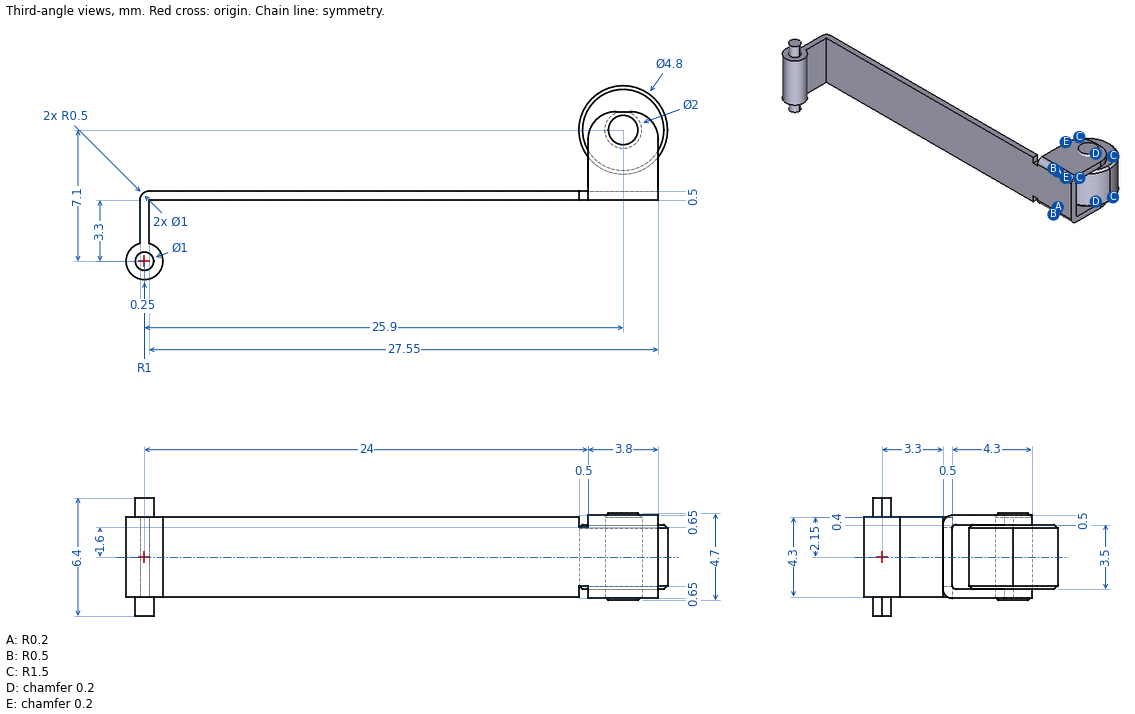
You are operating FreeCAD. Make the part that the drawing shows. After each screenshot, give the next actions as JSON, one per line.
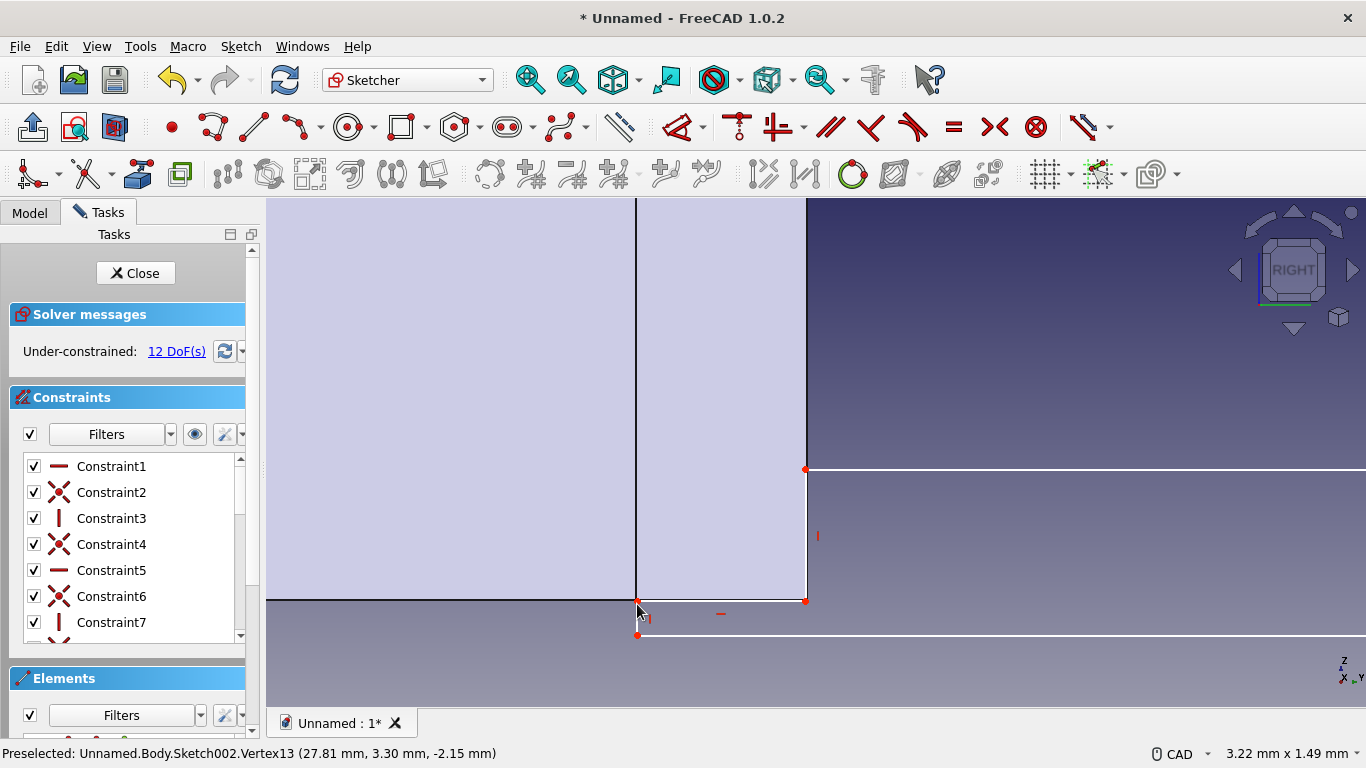
{"action": "scroll", "coordinate": [711, 601], "scroll_direction": "down", "scroll_amount": 8}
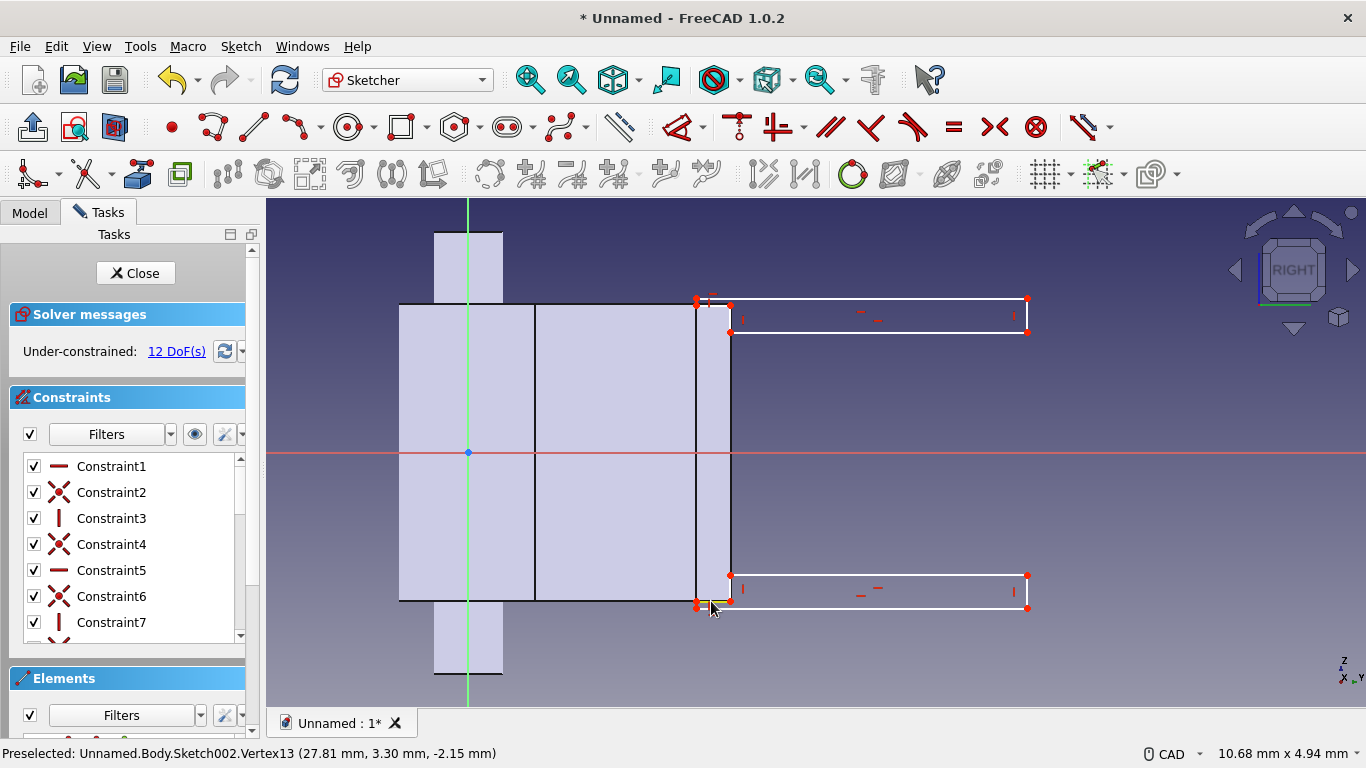
{"action": "scroll", "coordinate": [696, 306], "scroll_direction": "up", "scroll_amount": 3}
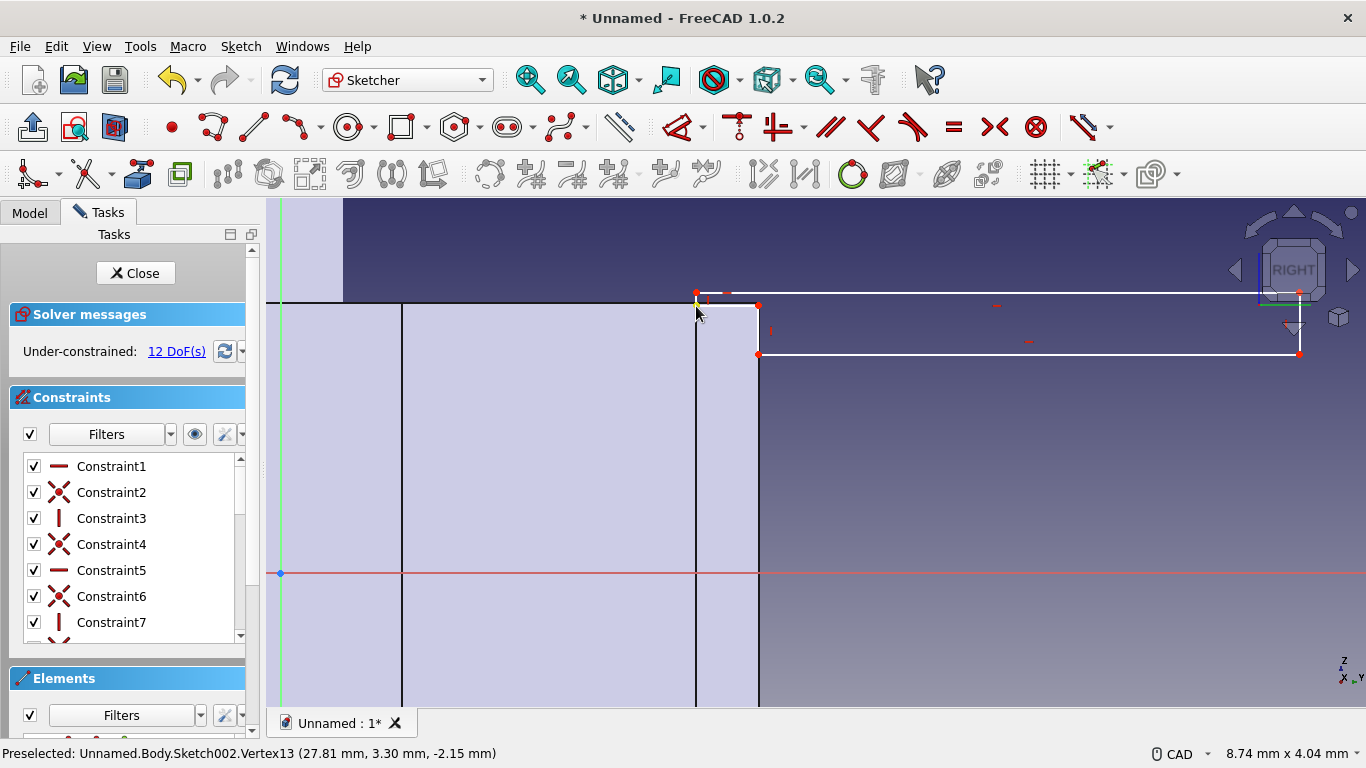
{"action": "left_click", "coordinate": [696, 306]}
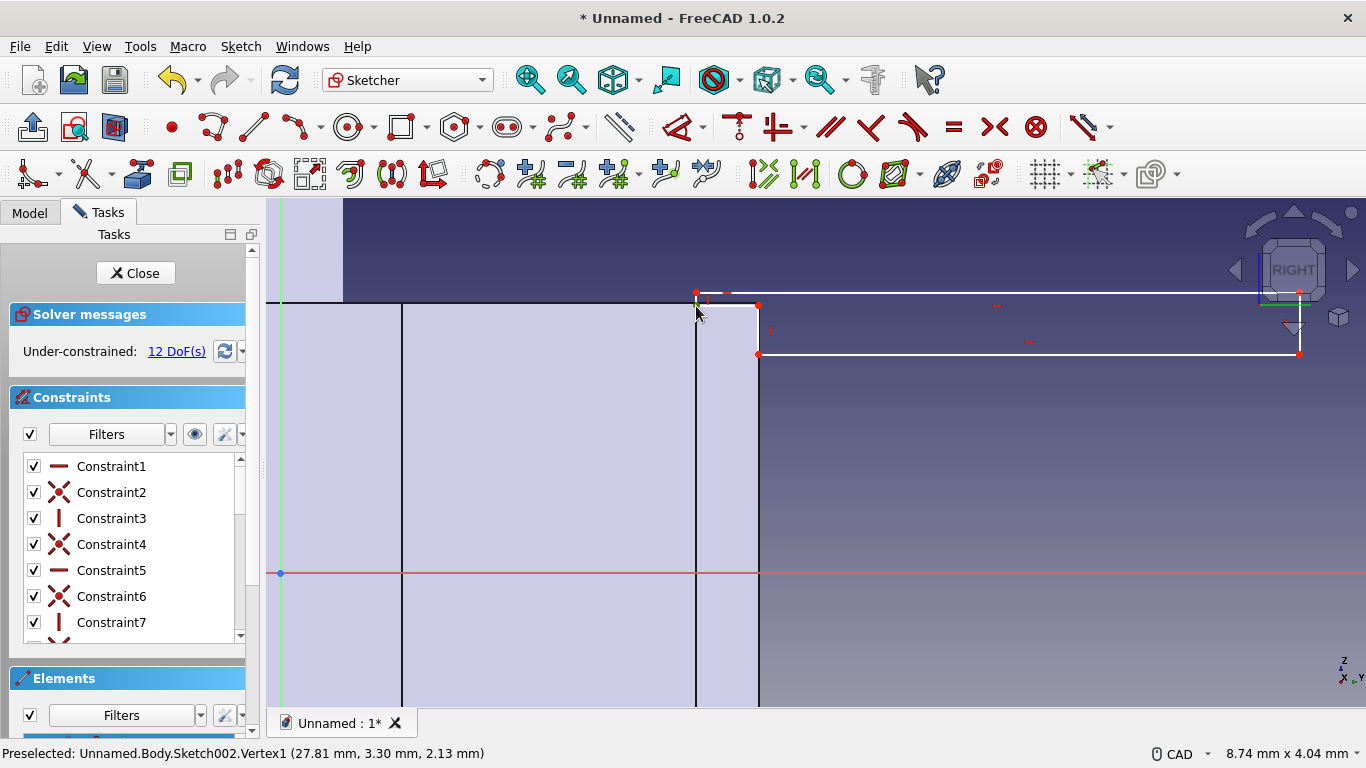
{"action": "scroll", "coordinate": [695, 305], "scroll_direction": "down", "scroll_amount": 3}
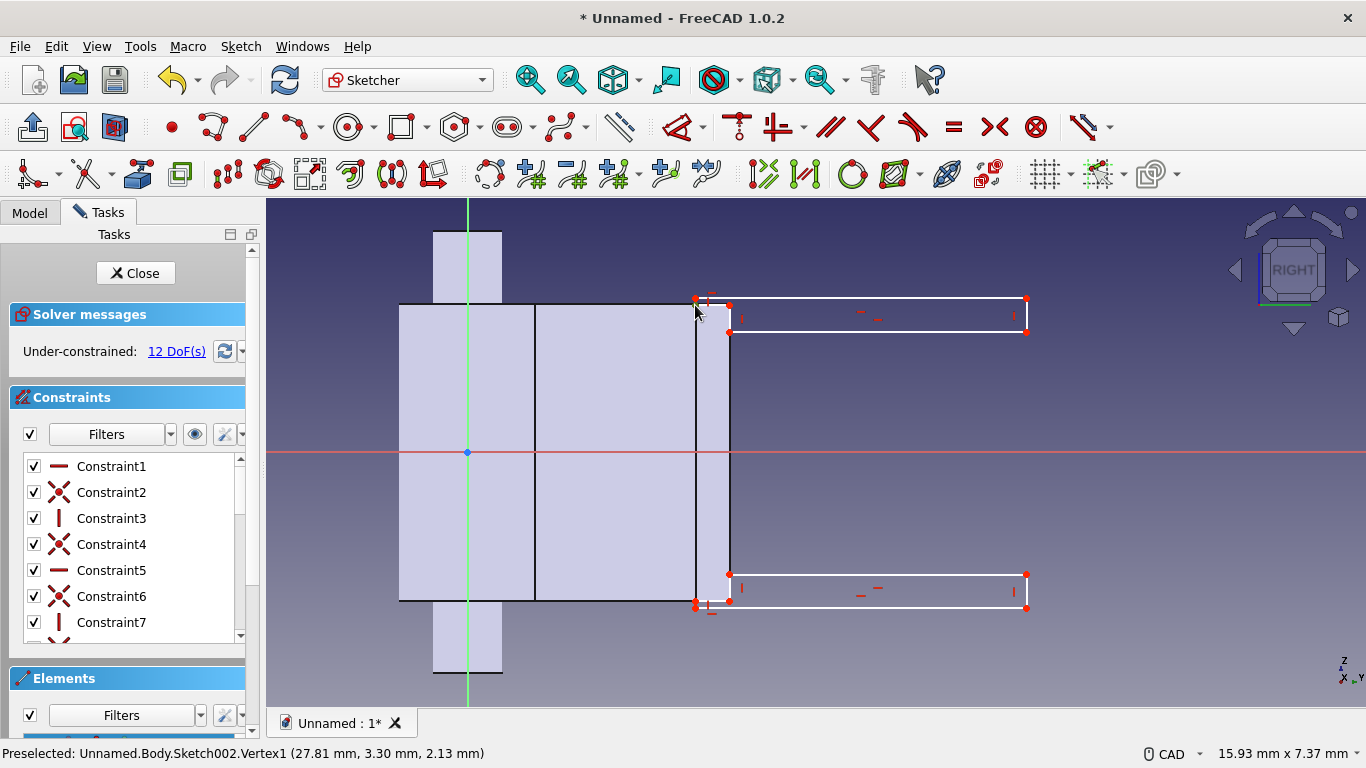
{"action": "scroll", "coordinate": [696, 601], "scroll_direction": "up", "scroll_amount": 3}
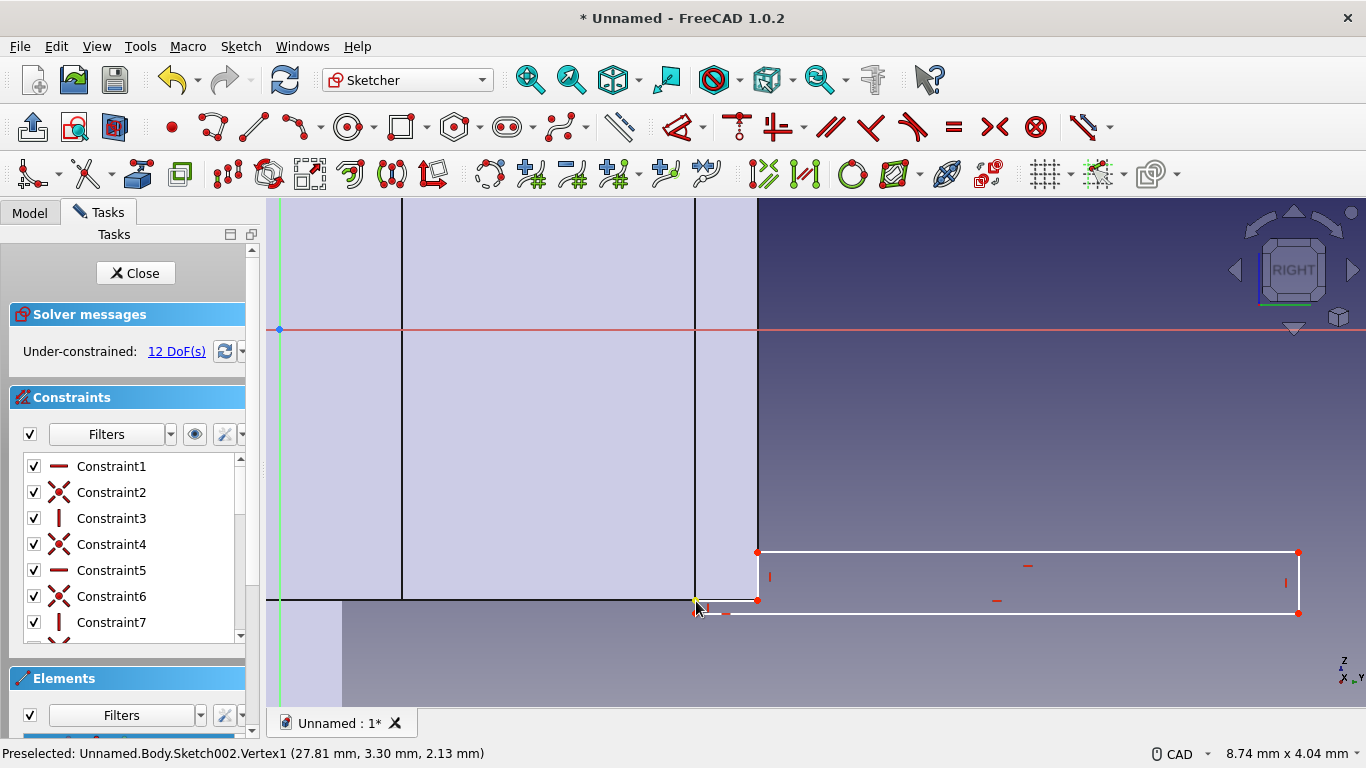
{"action": "left_click", "coordinate": [696, 601]}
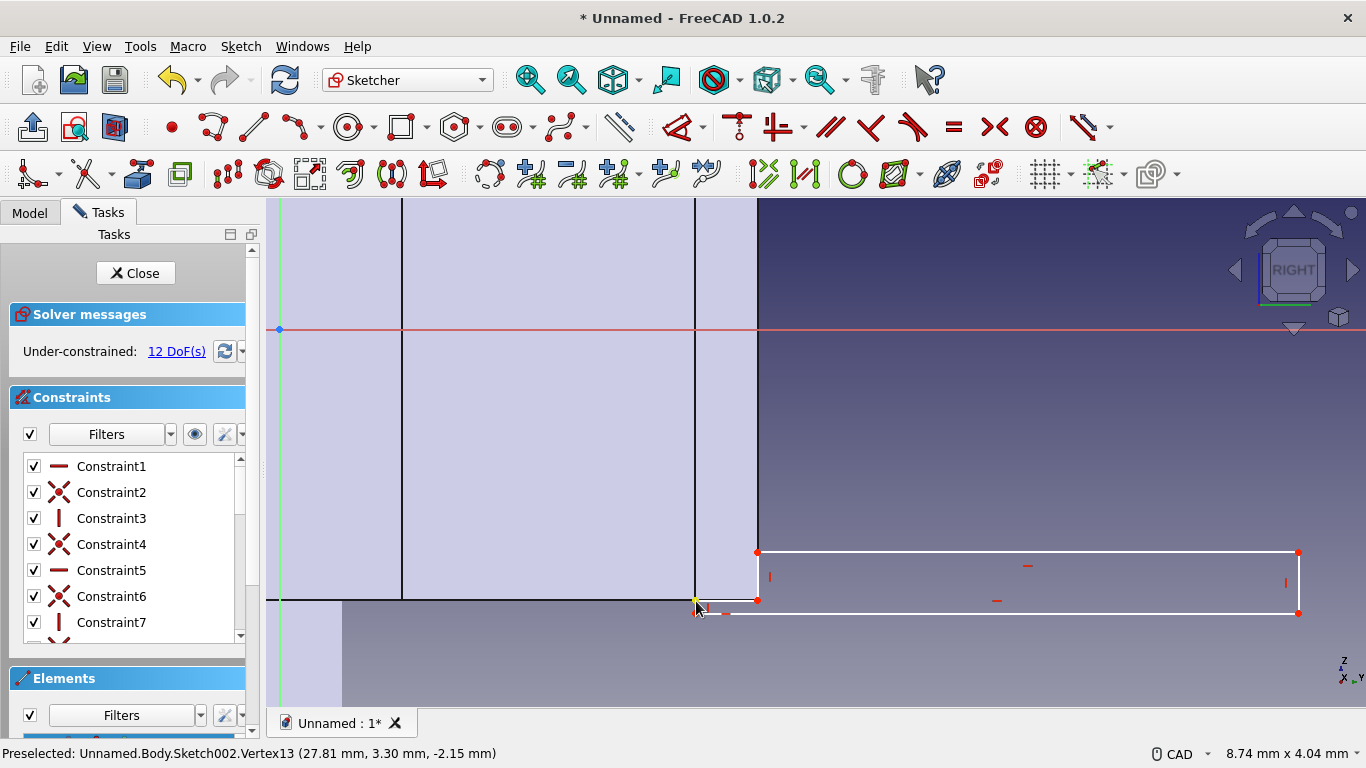
{"action": "left_click", "coordinate": [359, 330]}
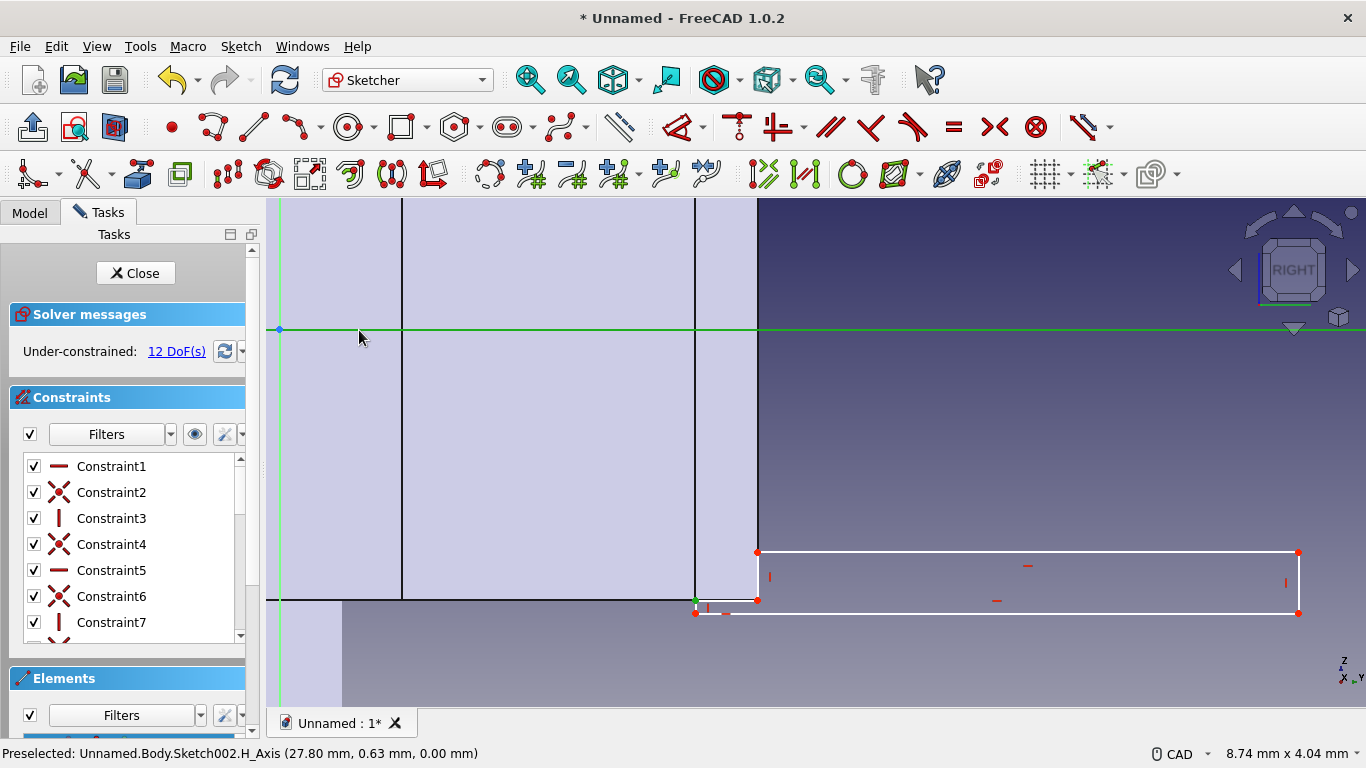
{"action": "key", "text": "s"}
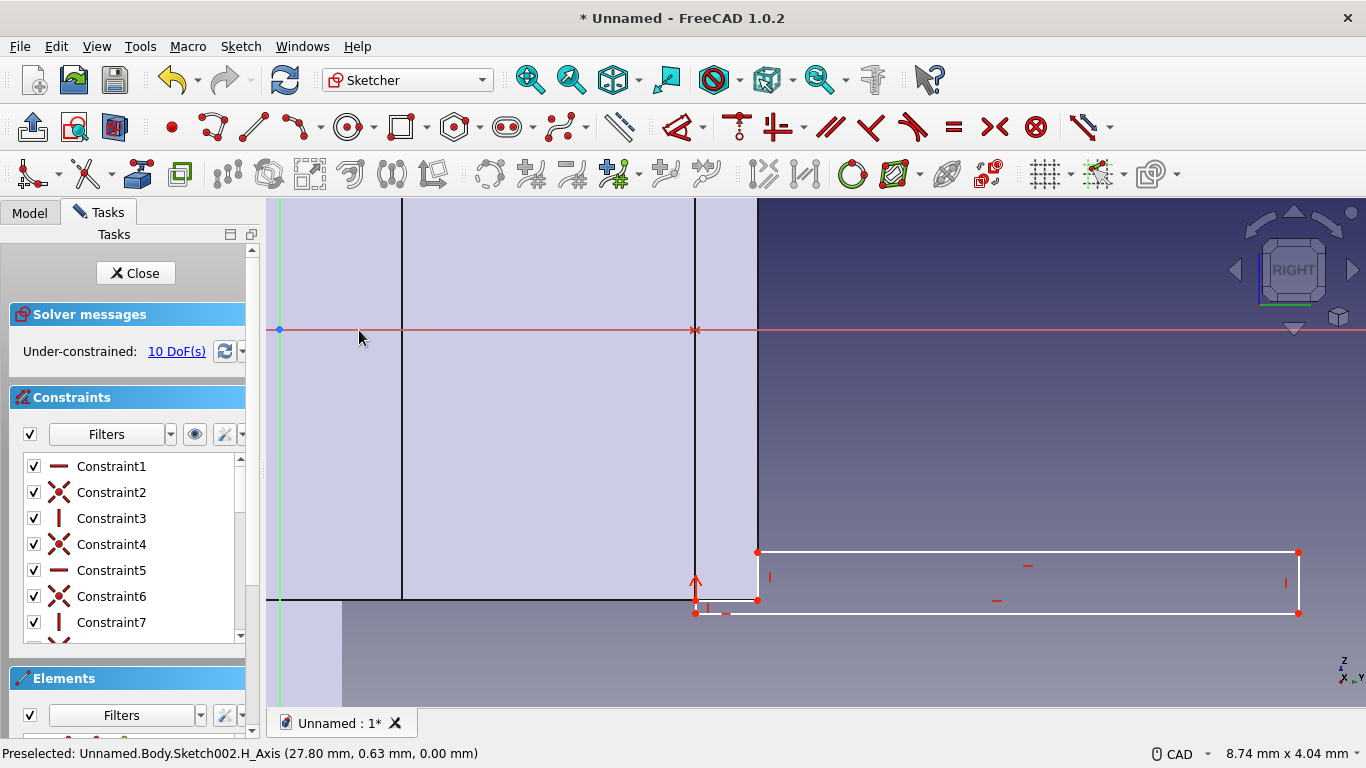
{"action": "scroll", "coordinate": [696, 602], "scroll_direction": "down", "scroll_amount": 3}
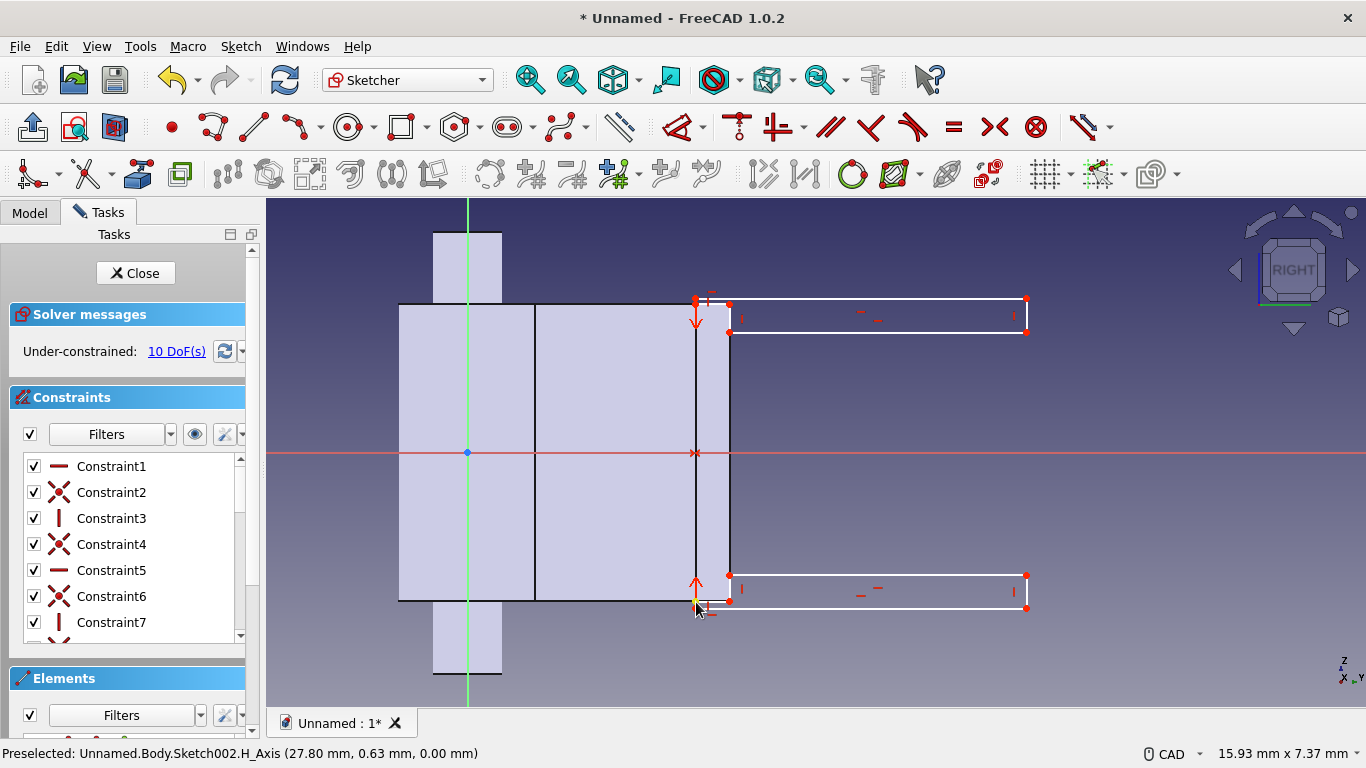
{"action": "left_click", "coordinate": [1027, 299]}